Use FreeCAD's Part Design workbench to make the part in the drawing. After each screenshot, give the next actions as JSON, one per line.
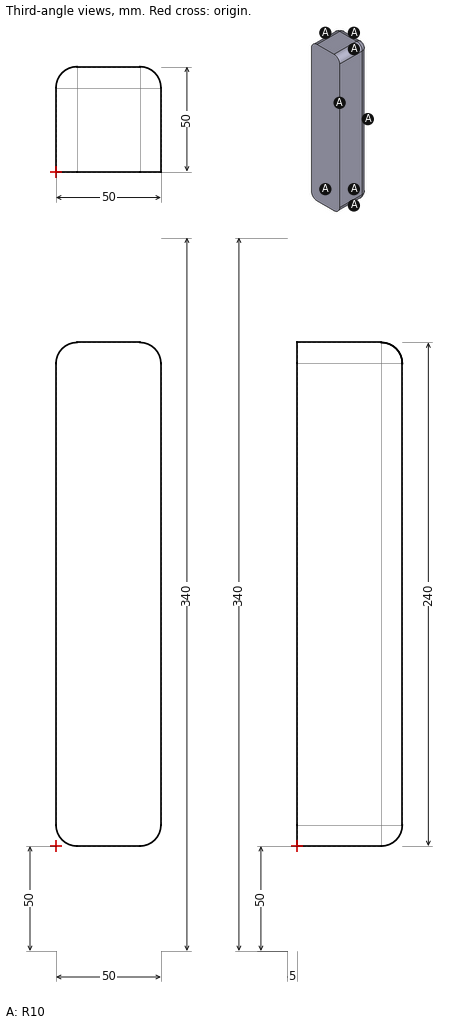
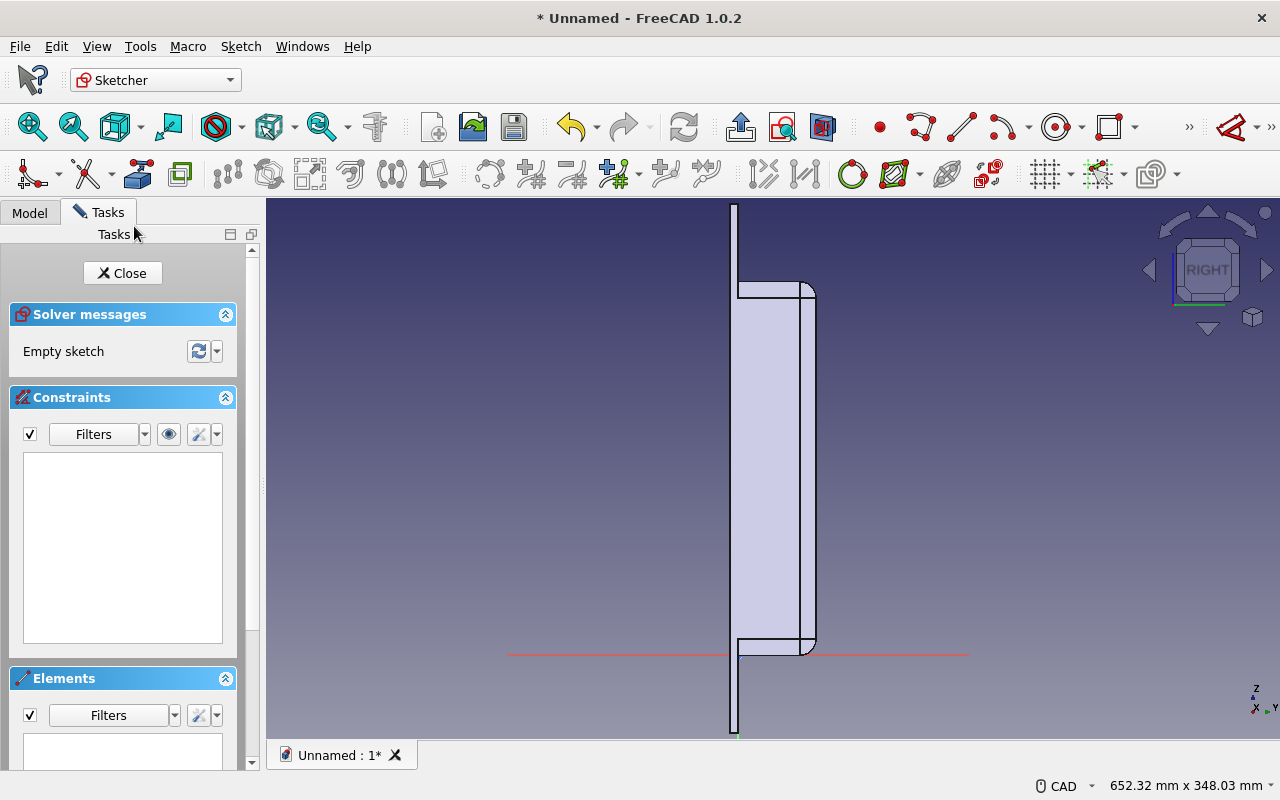
{"action": "left_click", "coordinate": [823, 128]}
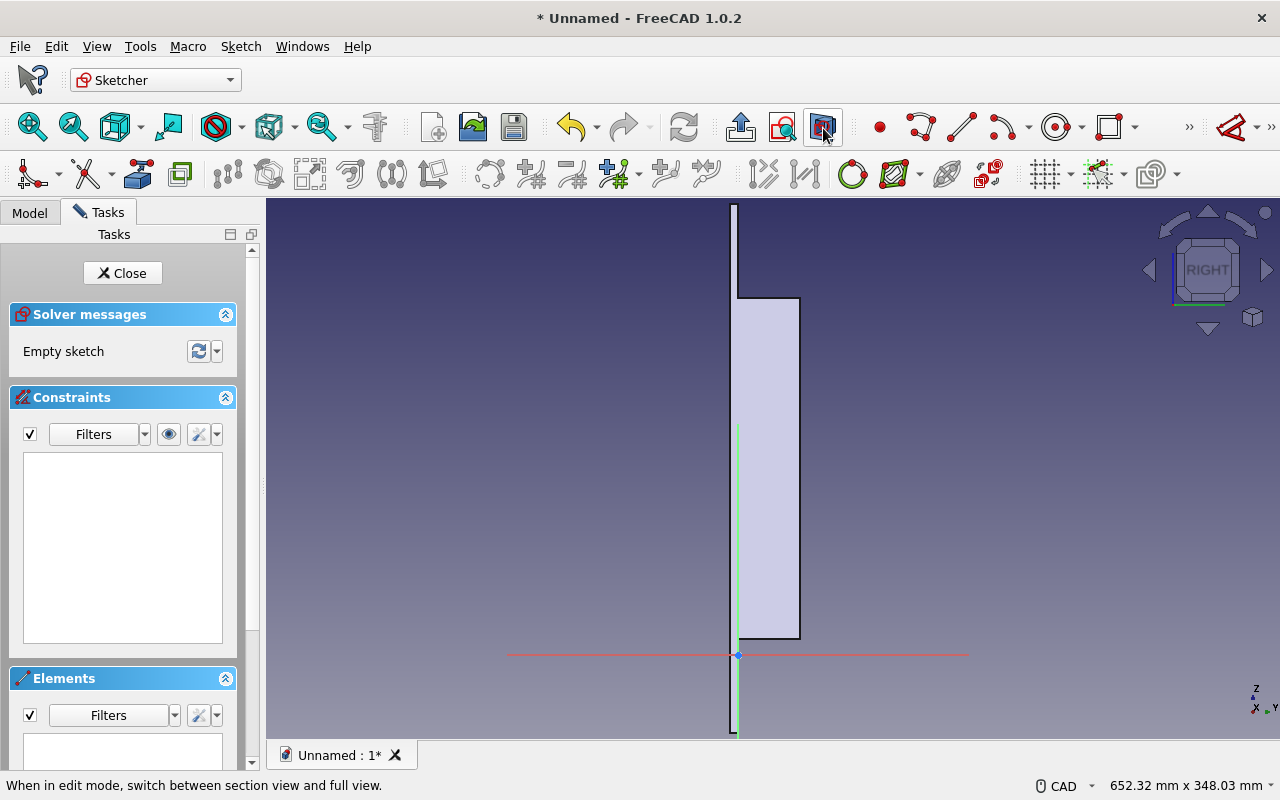
{"action": "scroll", "coordinate": [644, 469], "scroll_direction": "down", "scroll_amount": 2}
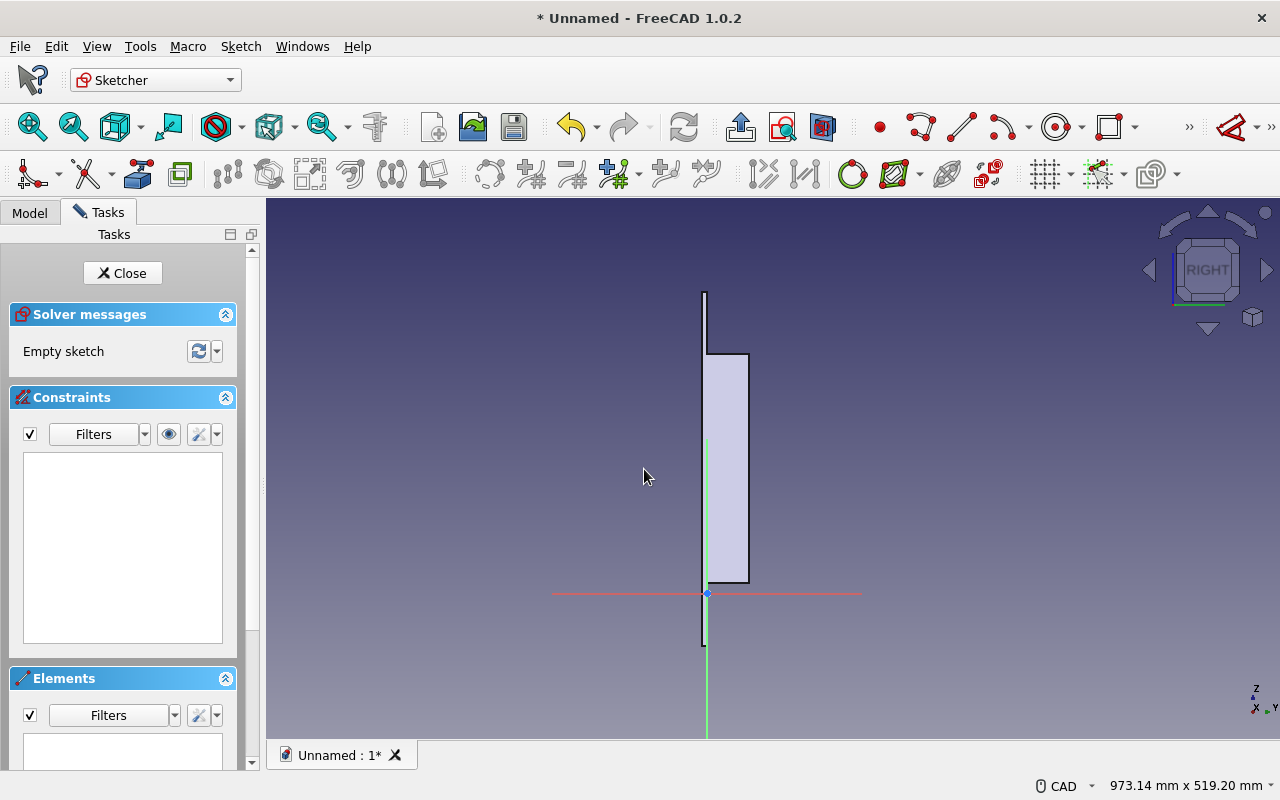
{"action": "left_click", "coordinate": [1108, 128]}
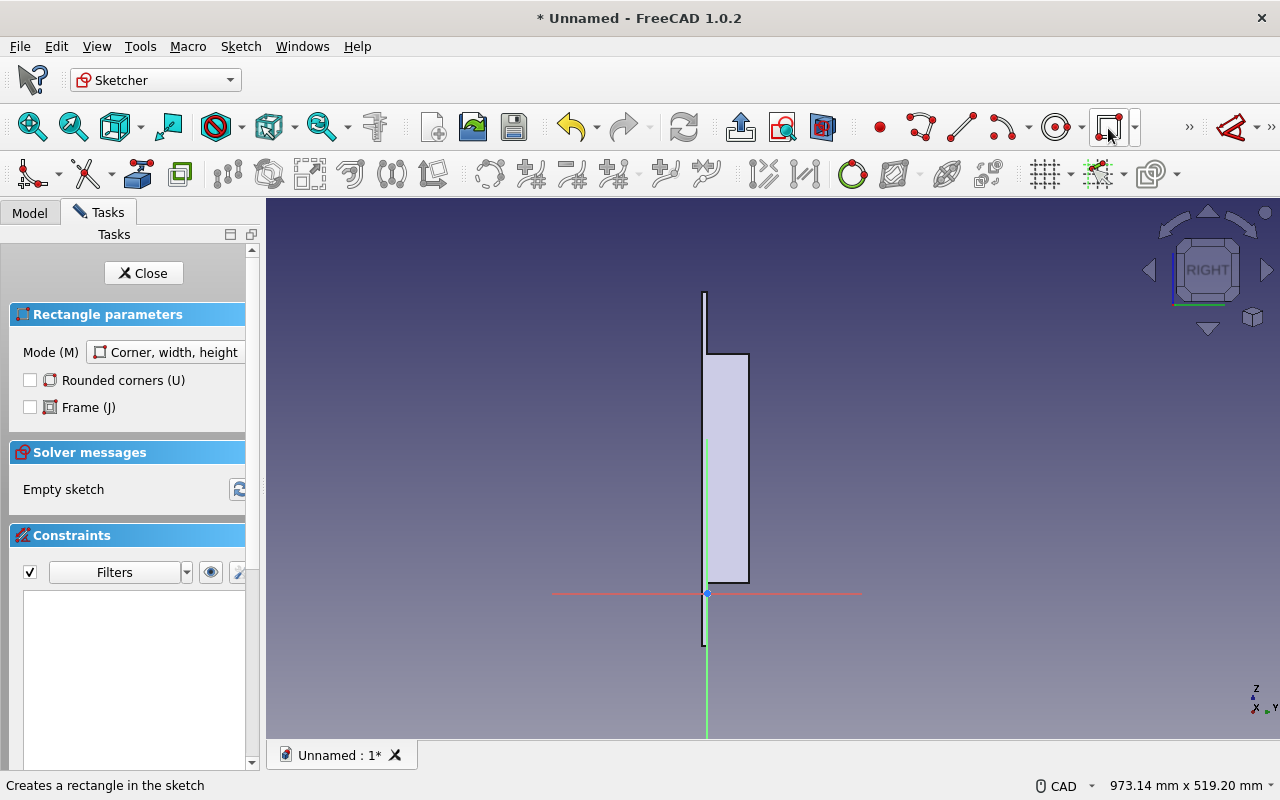
{"action": "scroll", "coordinate": [702, 292], "scroll_direction": "up", "scroll_amount": 6}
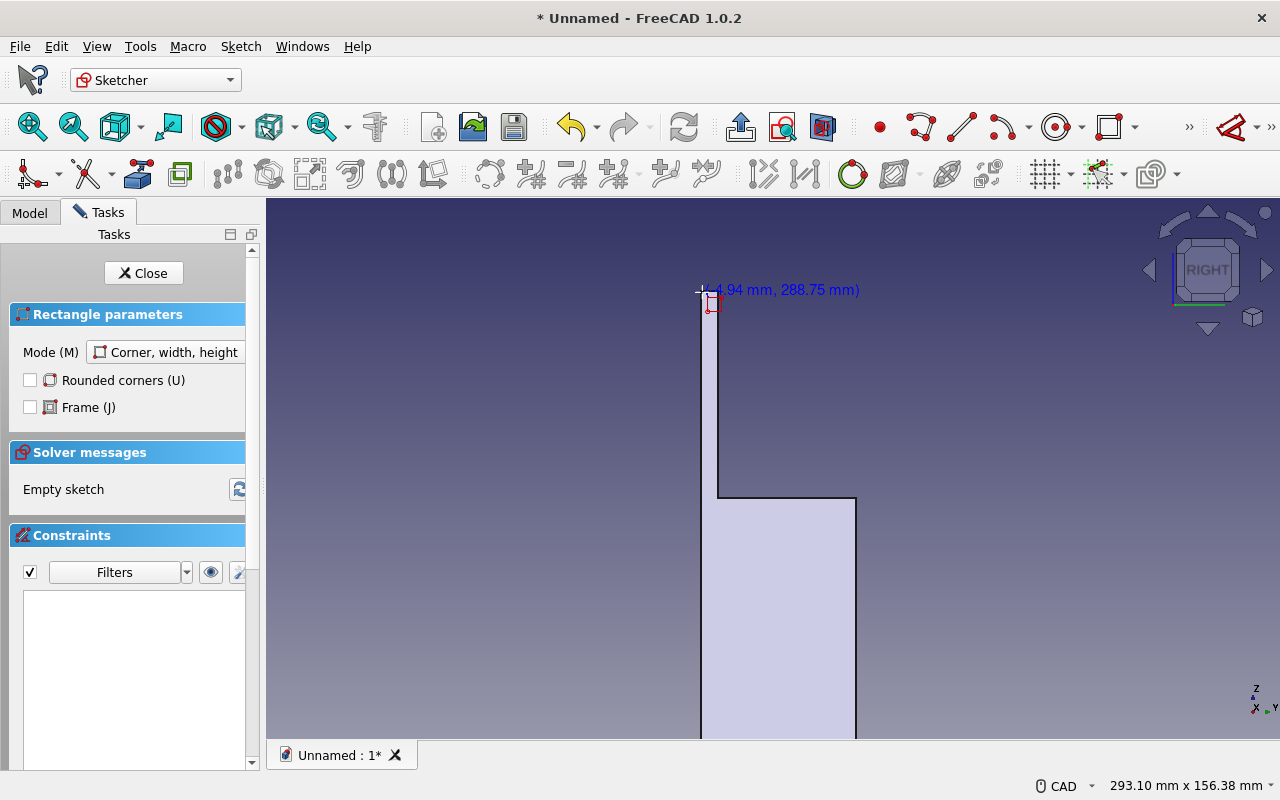
{"action": "left_click", "coordinate": [701, 291]}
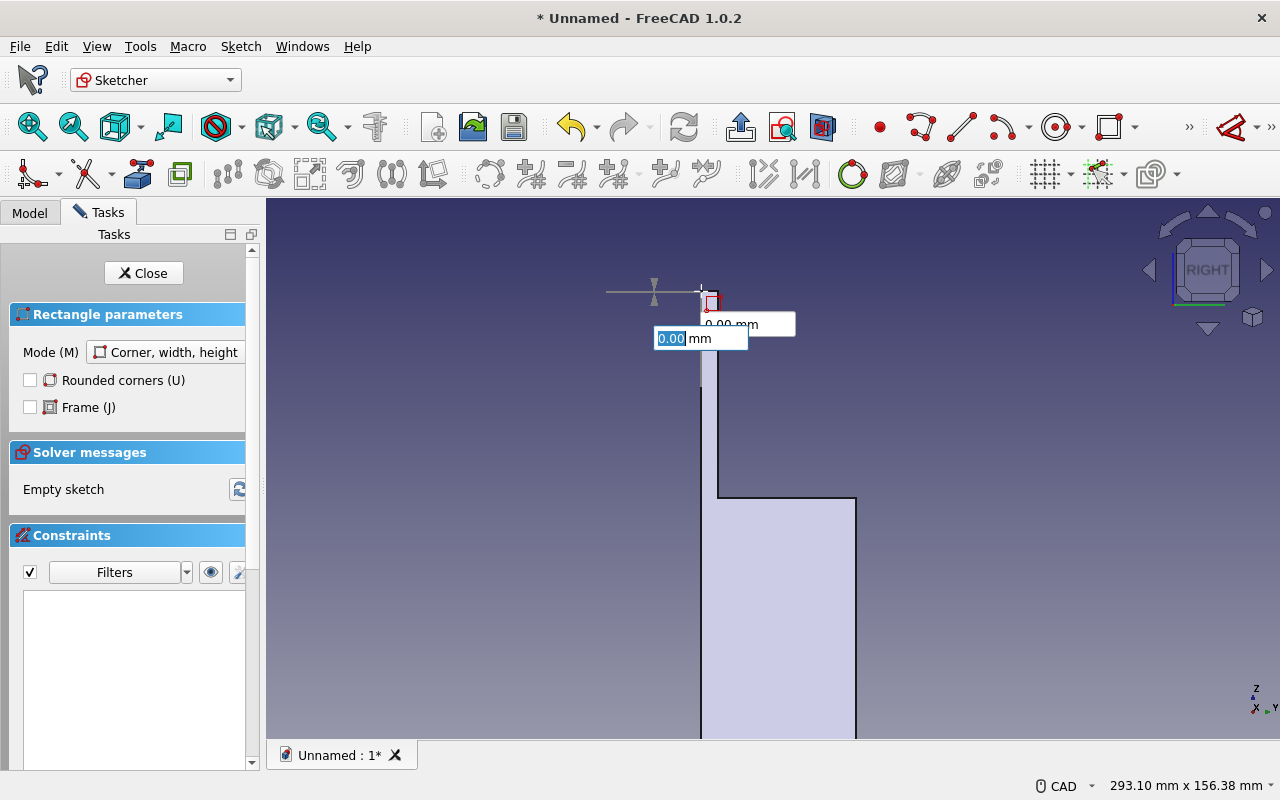
{"action": "scroll", "coordinate": [702, 292], "scroll_direction": "down", "scroll_amount": 6}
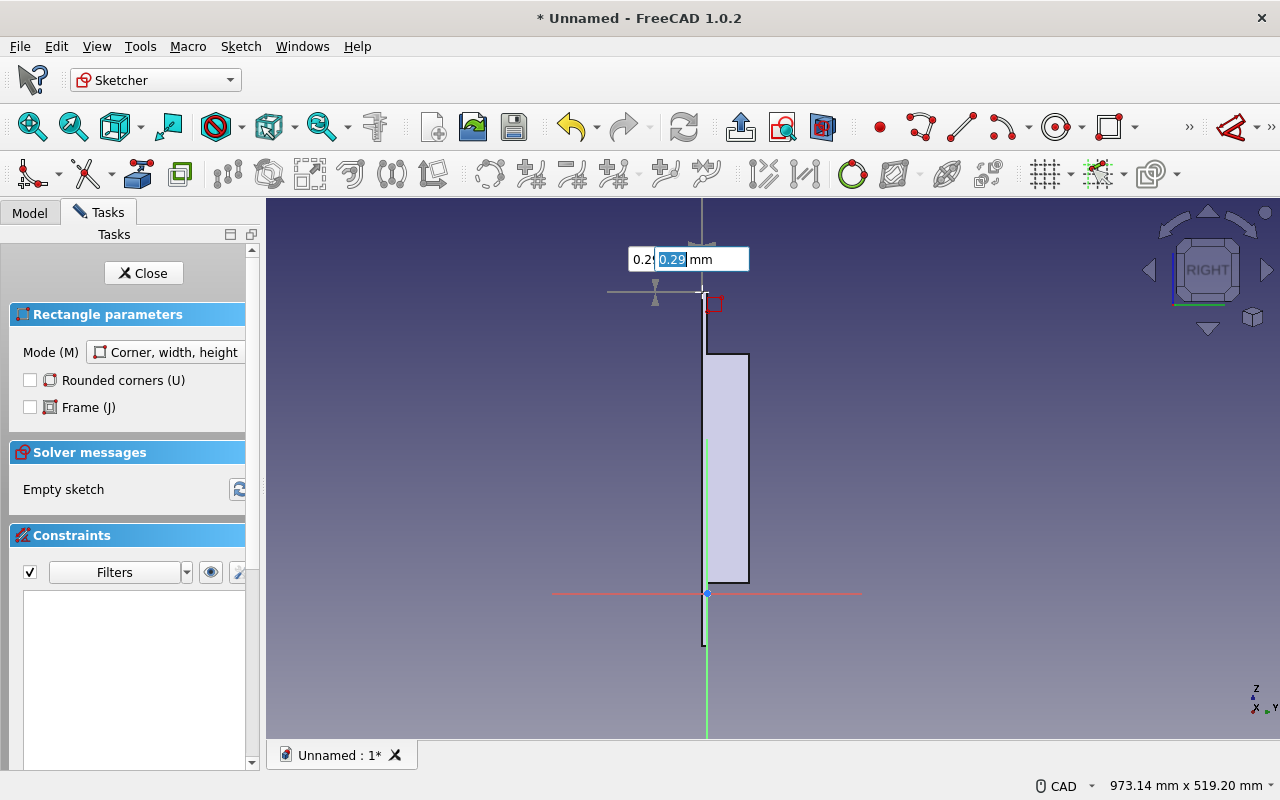
{"action": "left_click", "coordinate": [707, 646]}
{"action": "key", "text": "Escape"}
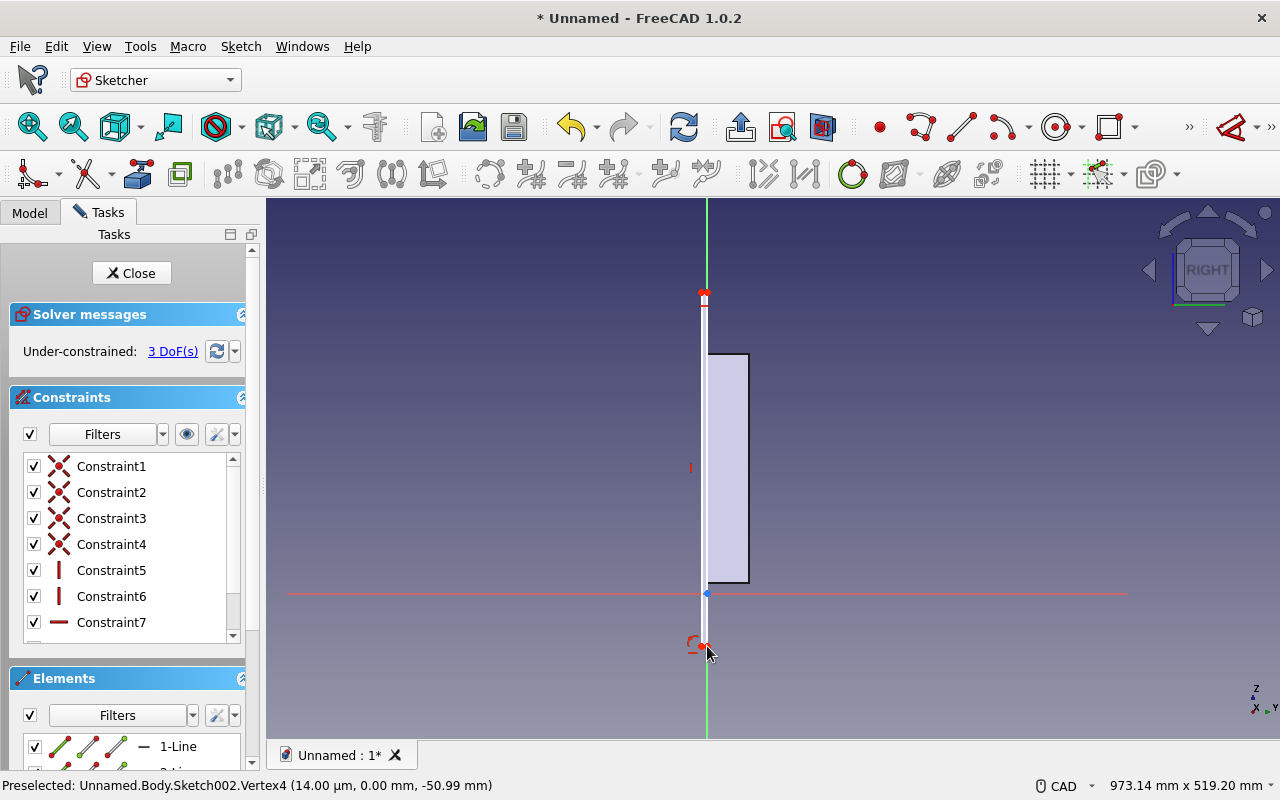
{"action": "left_click", "coordinate": [1230, 128]}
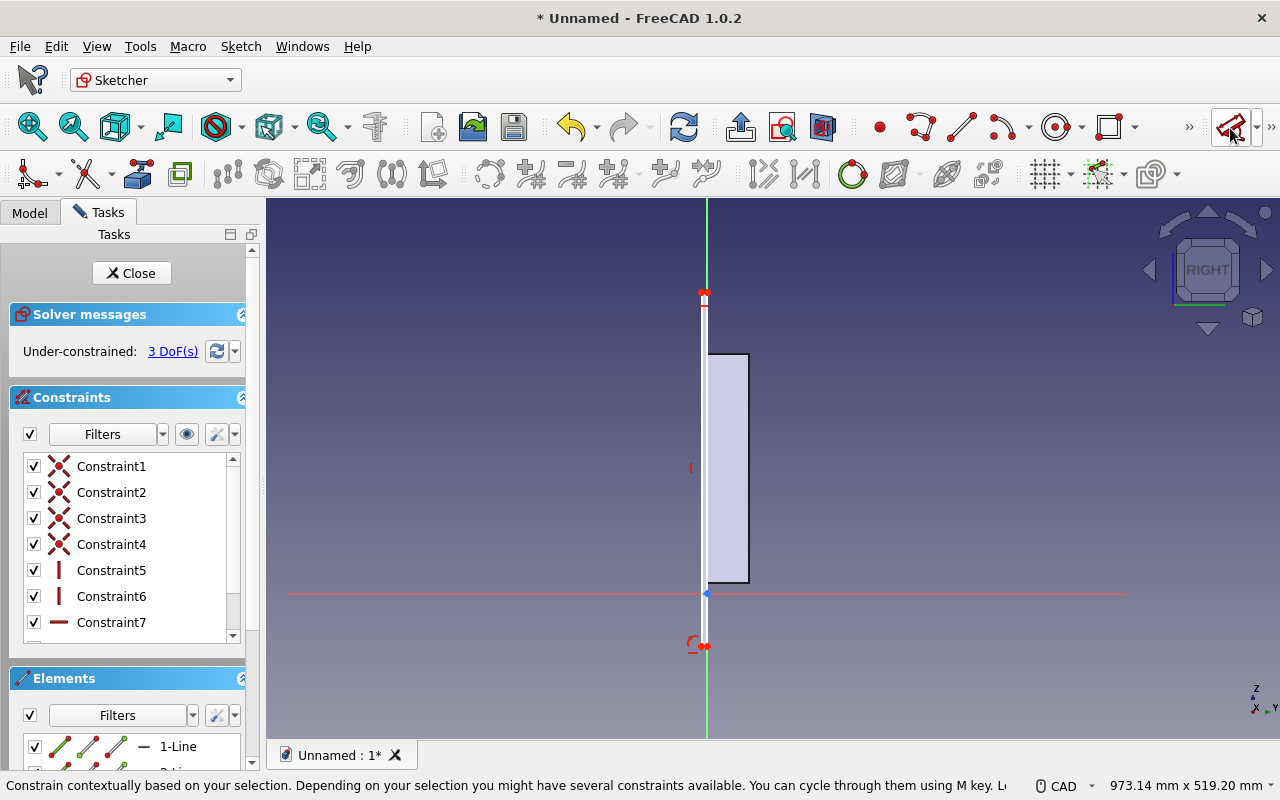
{"action": "scroll", "coordinate": [705, 647], "scroll_direction": "up", "scroll_amount": 11}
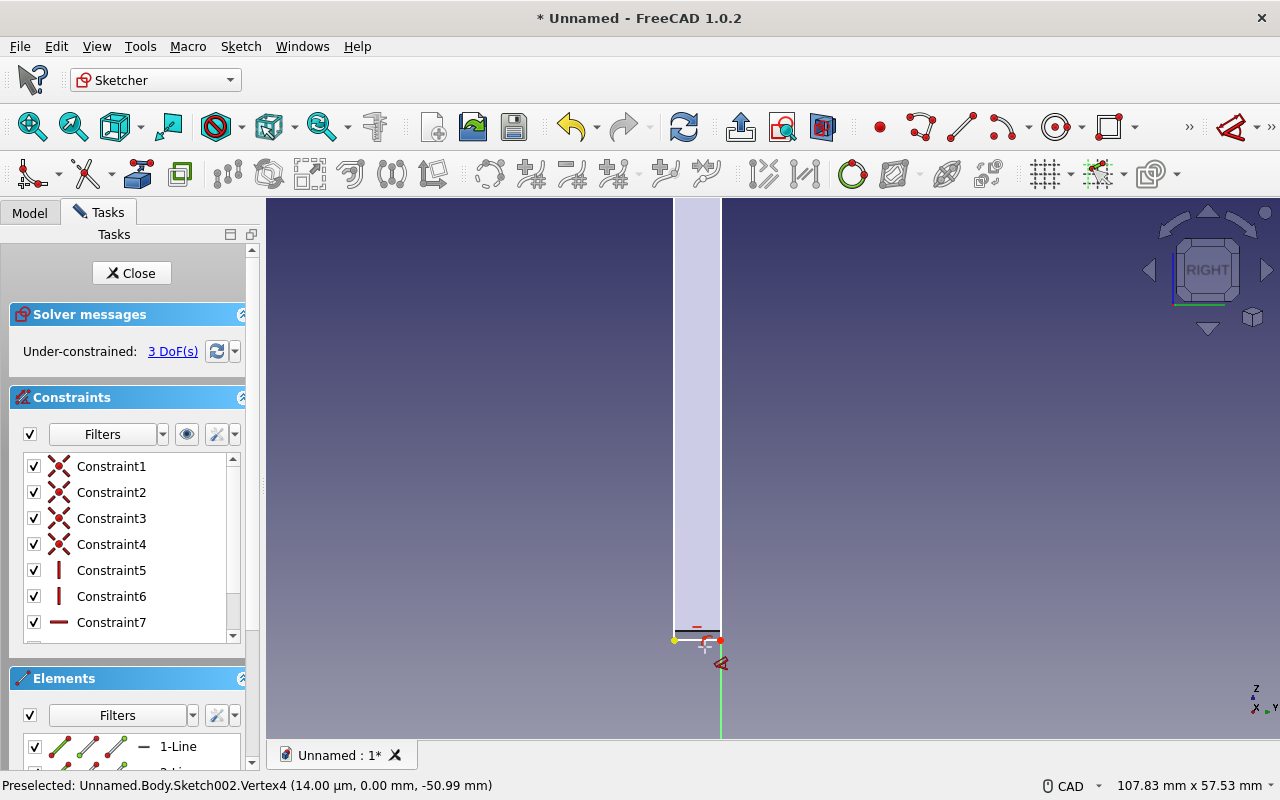
{"action": "left_click", "coordinate": [698, 640]}
{"action": "left_click", "coordinate": [698, 674]}